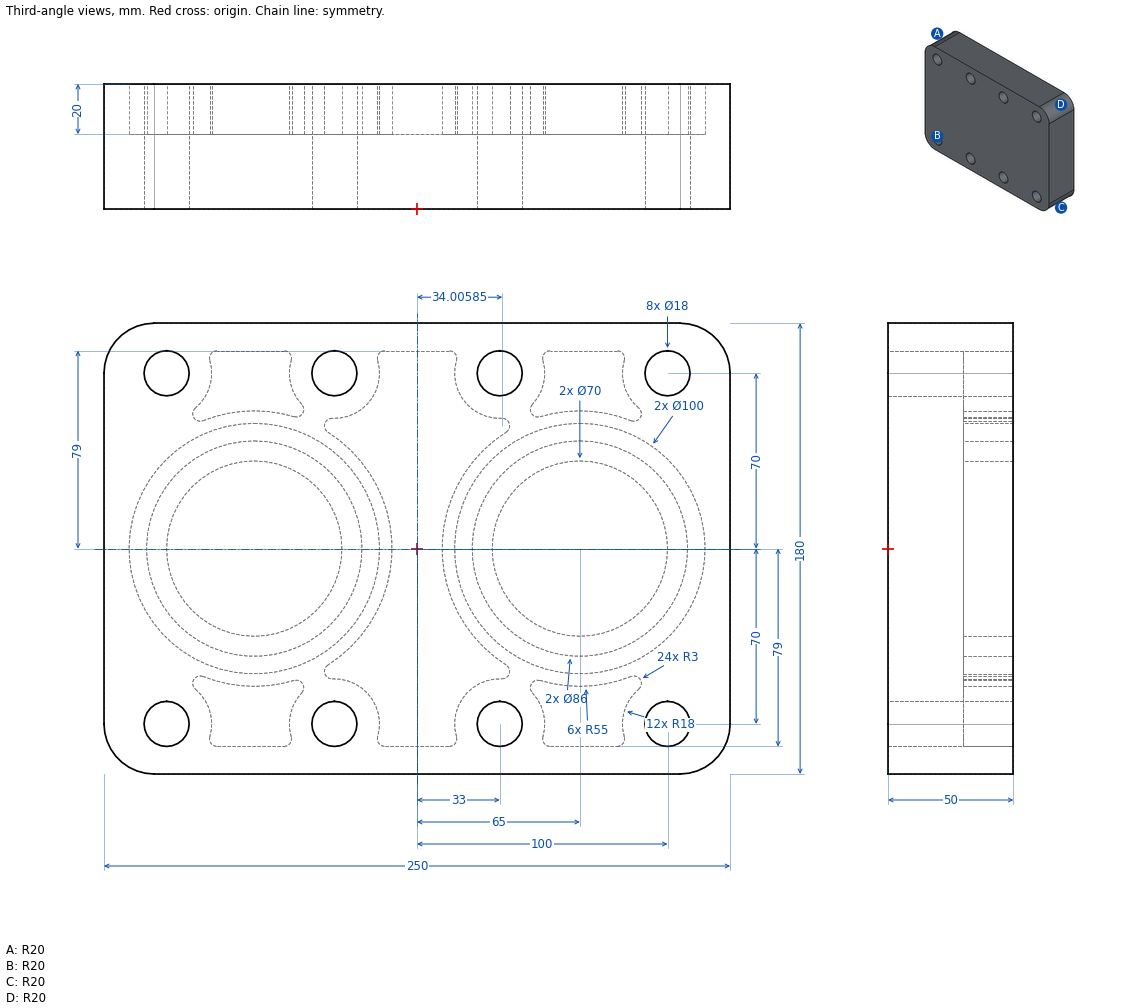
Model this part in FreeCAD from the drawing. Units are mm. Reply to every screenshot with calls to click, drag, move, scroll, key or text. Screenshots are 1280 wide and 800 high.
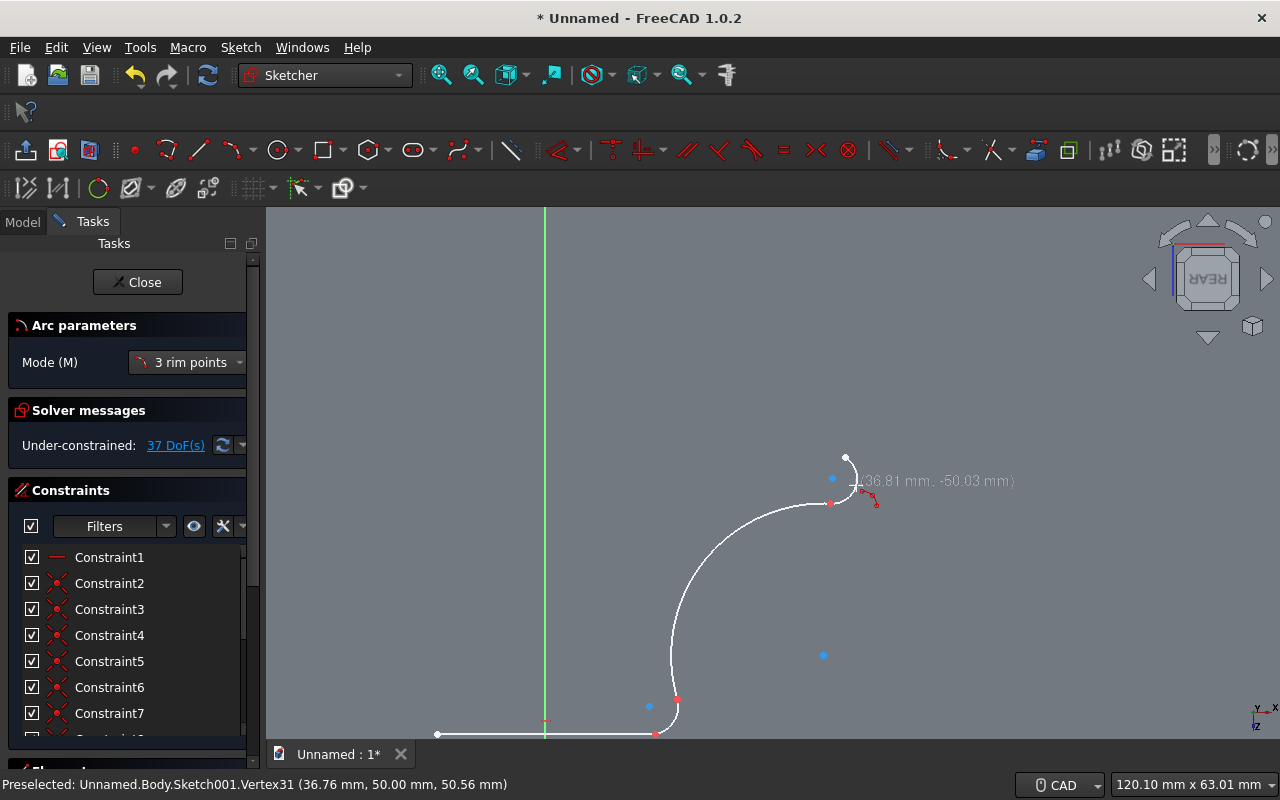
click(845, 457)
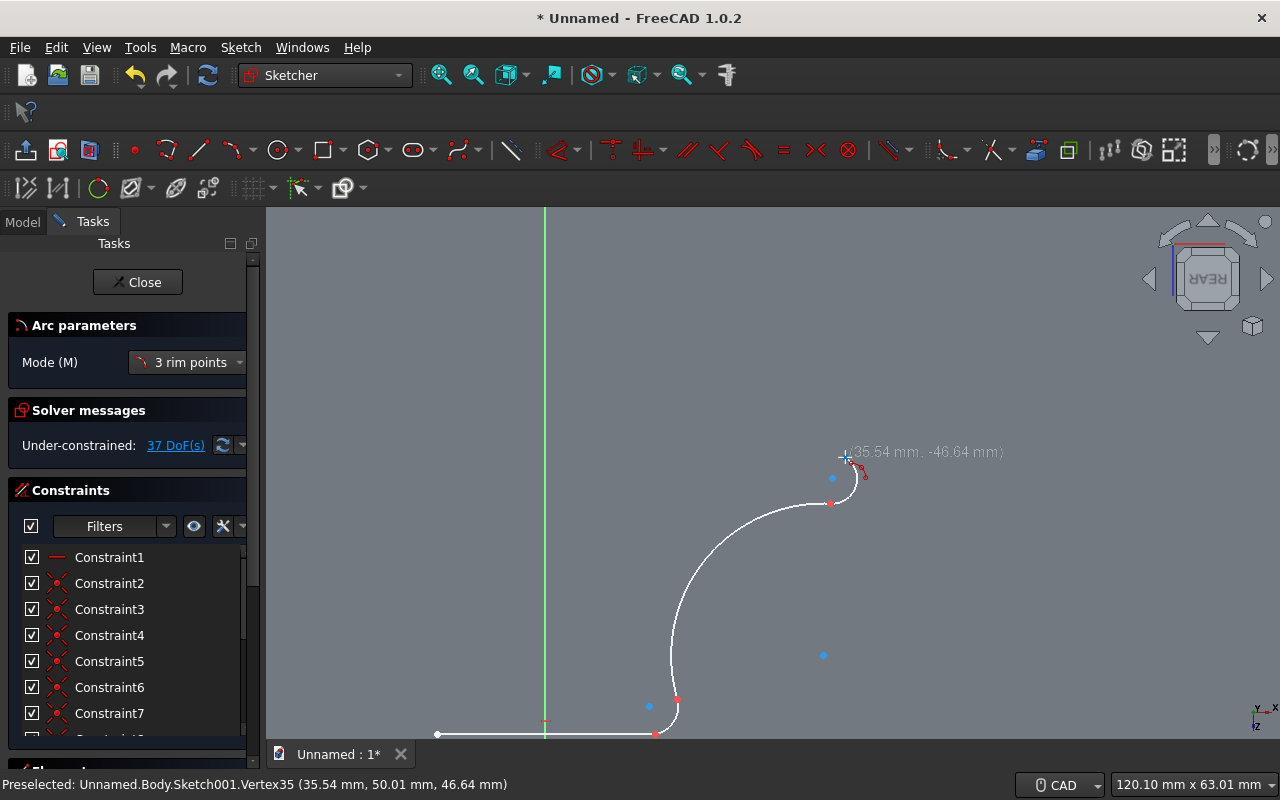
scroll(757, 607, down, 7)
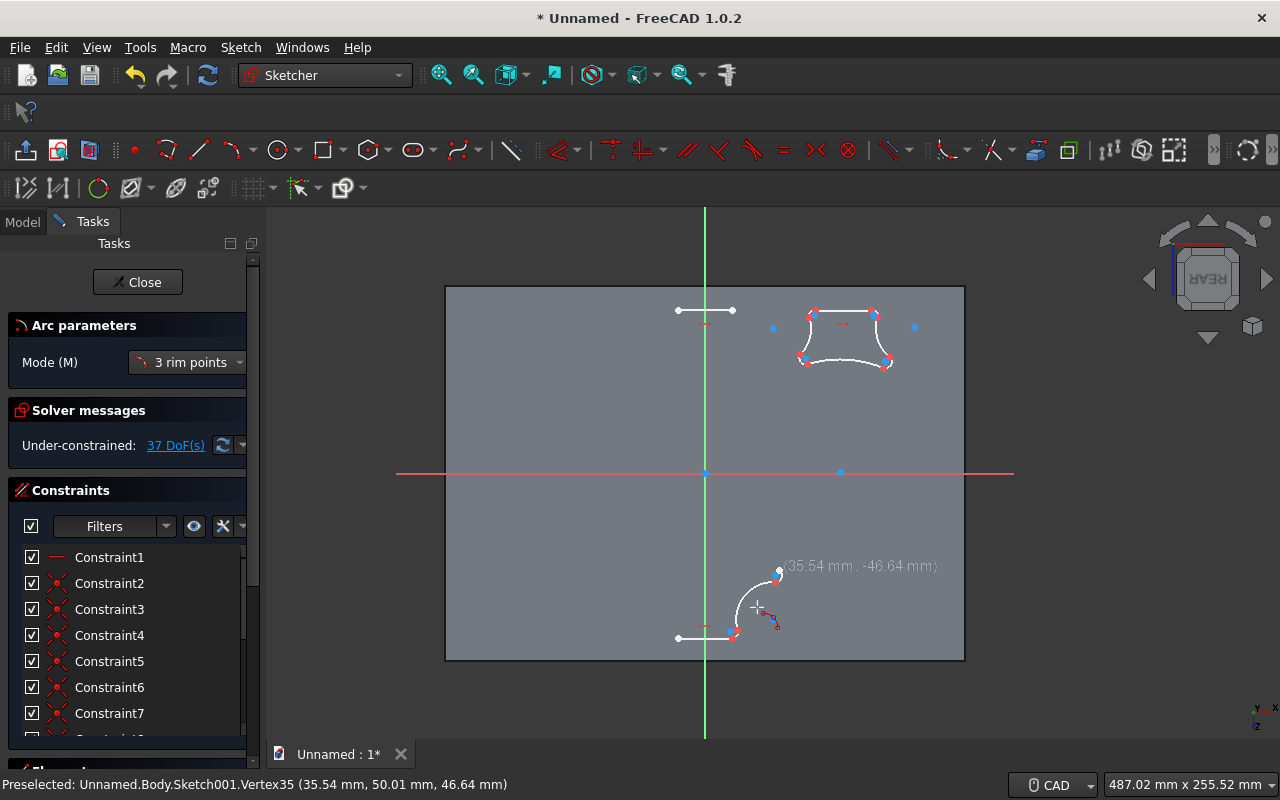
click(779, 377)
click(728, 451)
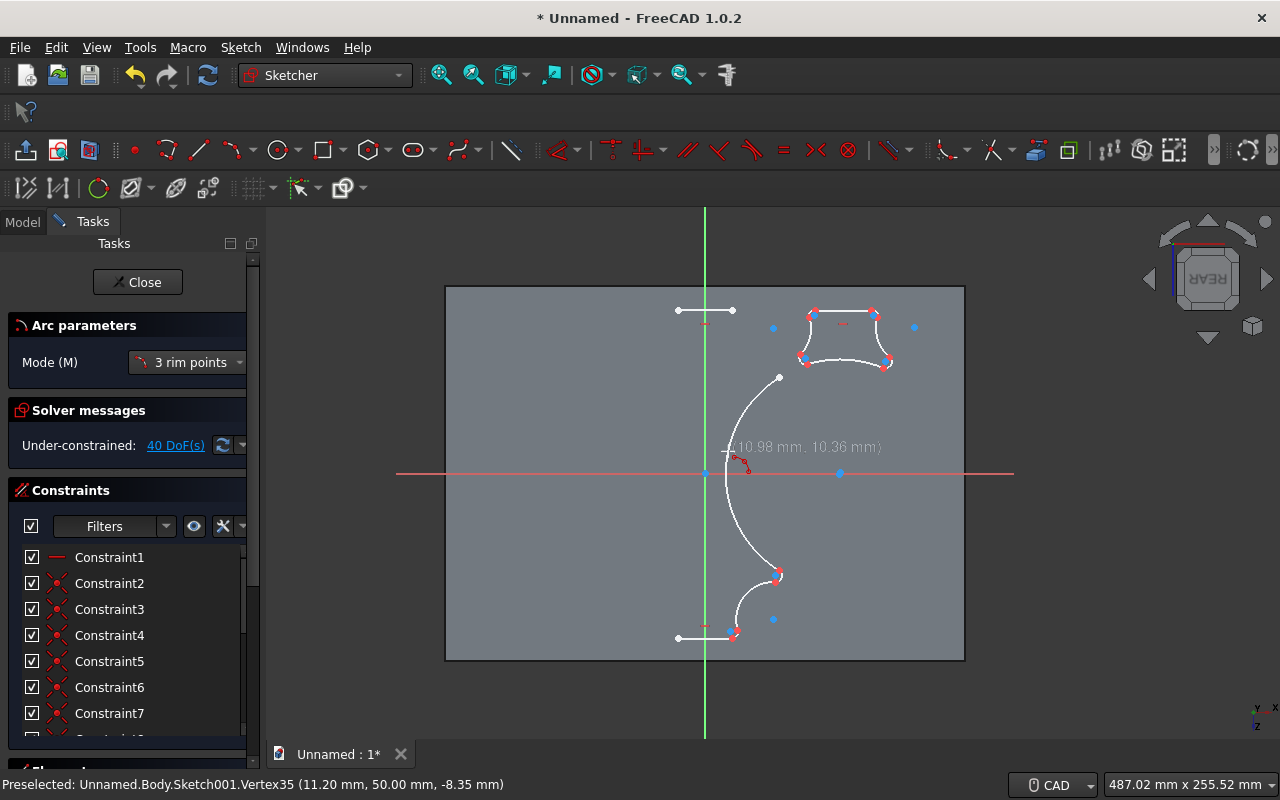
click(779, 378)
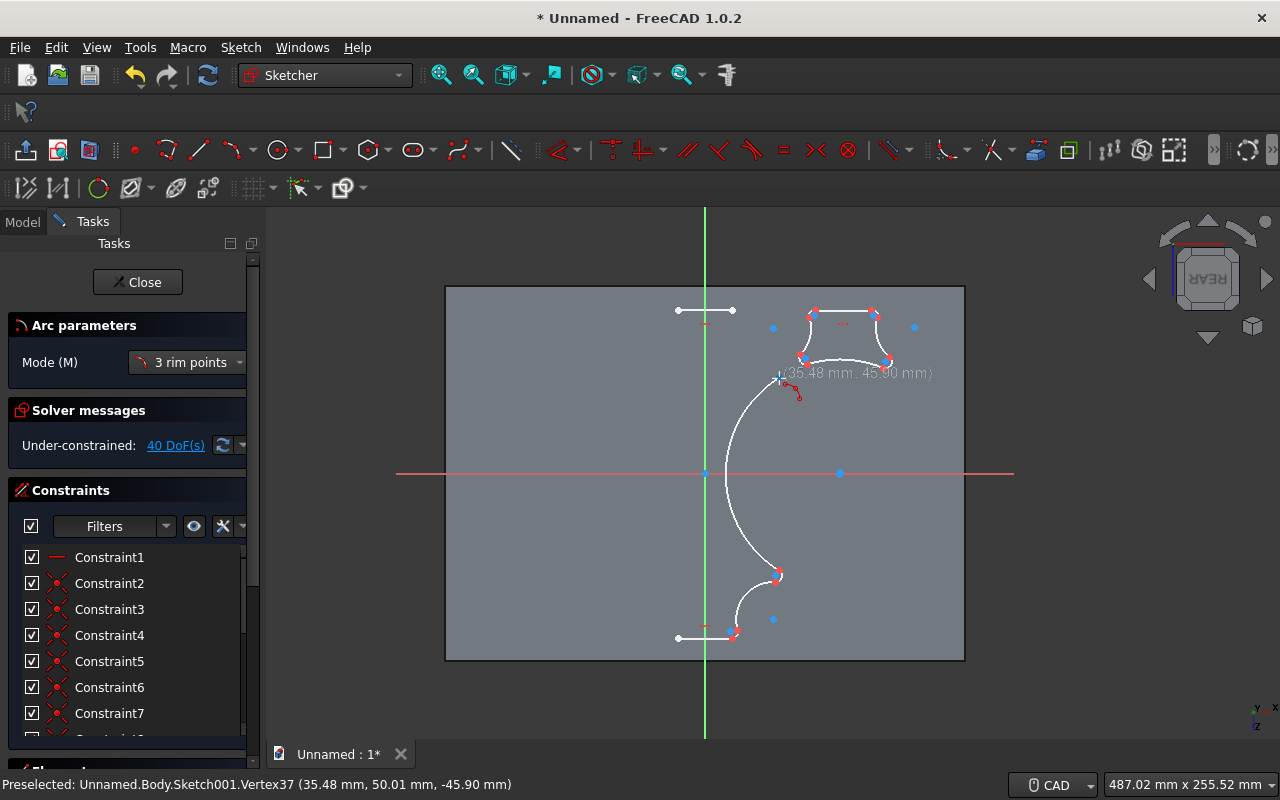
scroll(776, 365, up, 2)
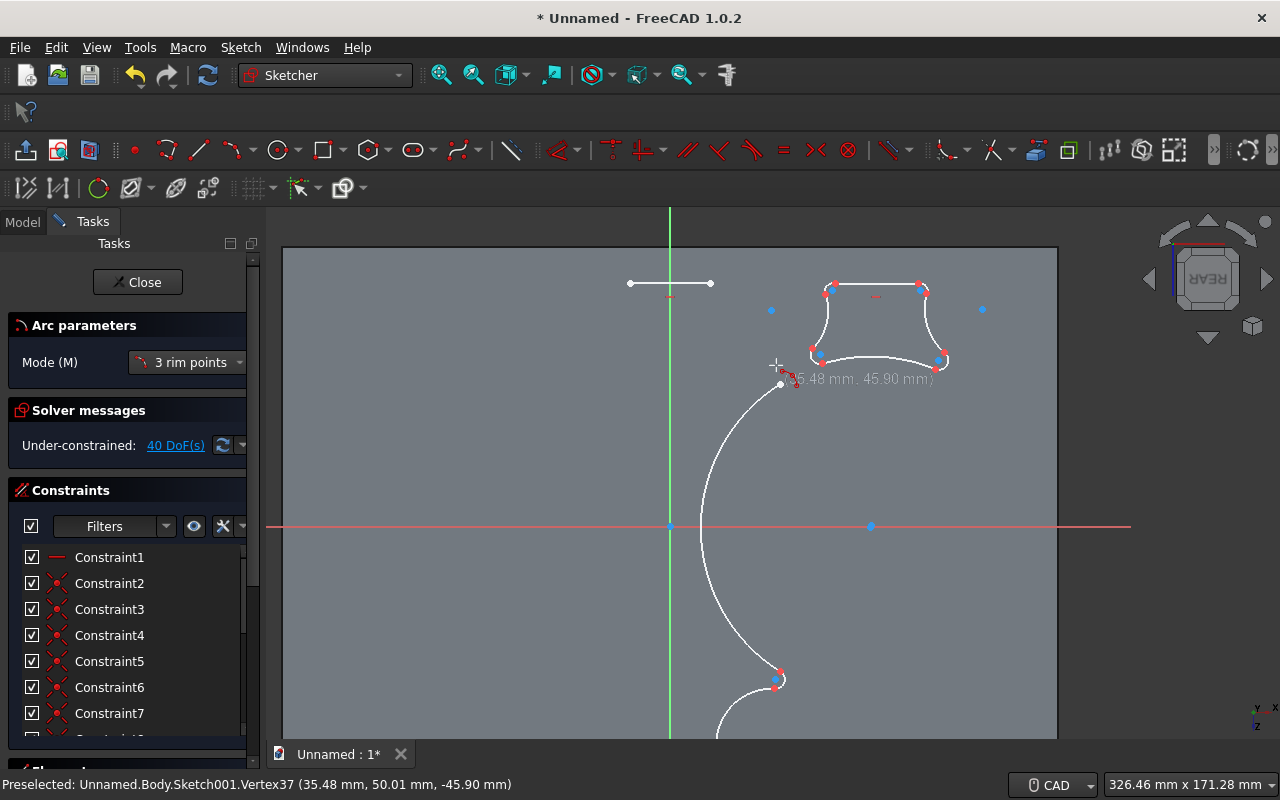
click(775, 365)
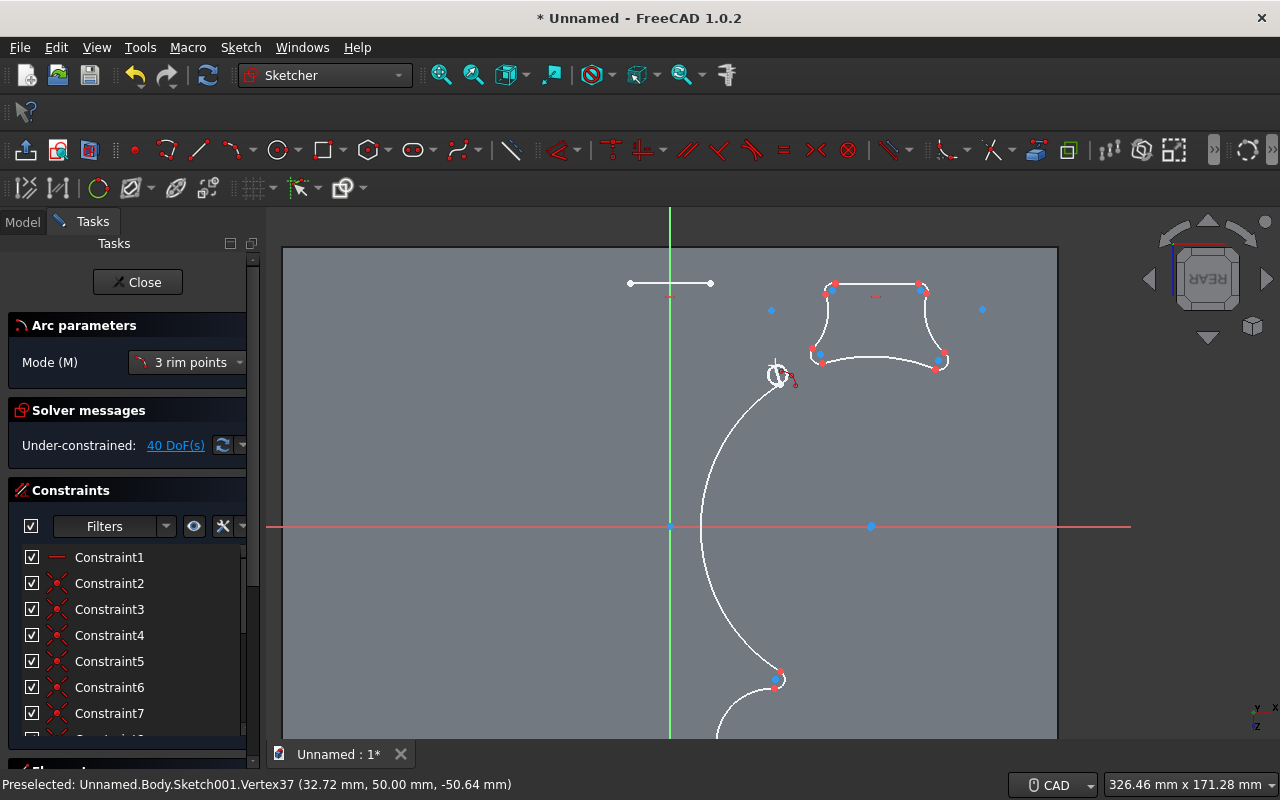
scroll(785, 372, up, 5)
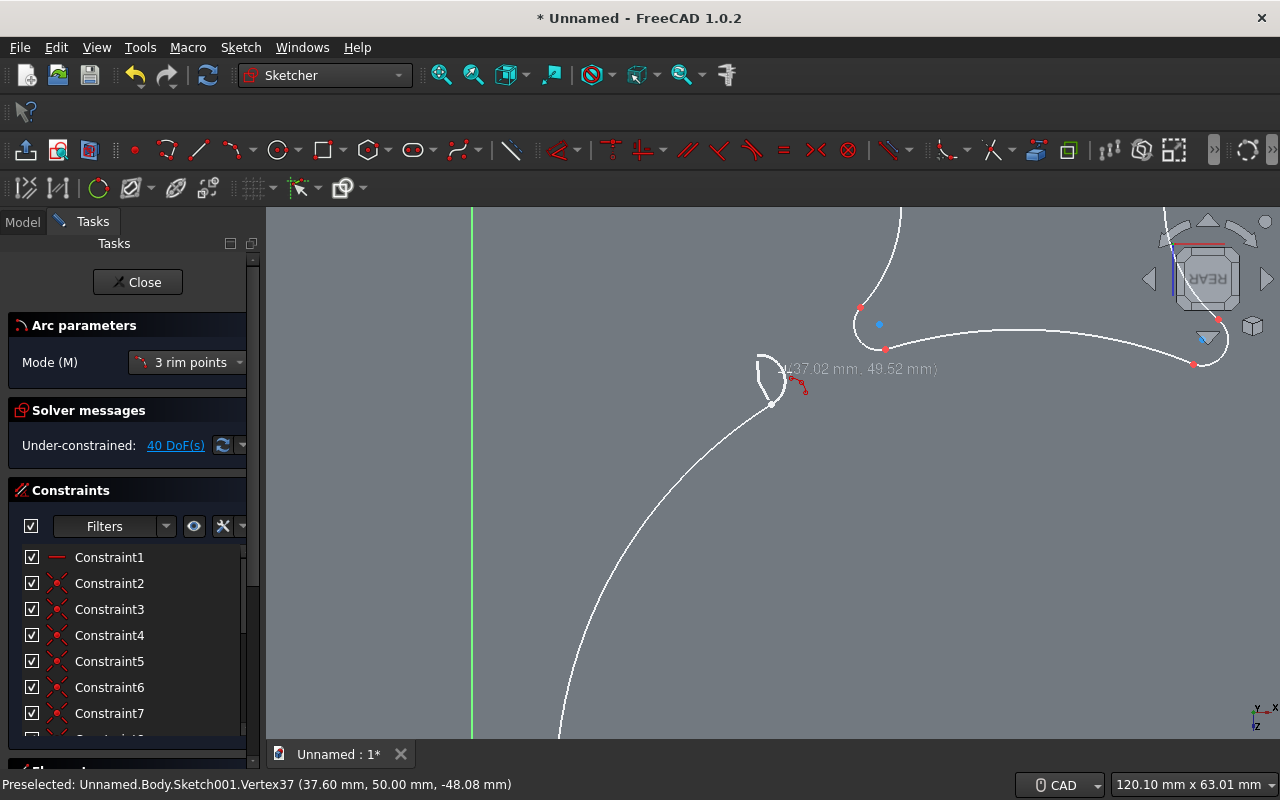
click(783, 371)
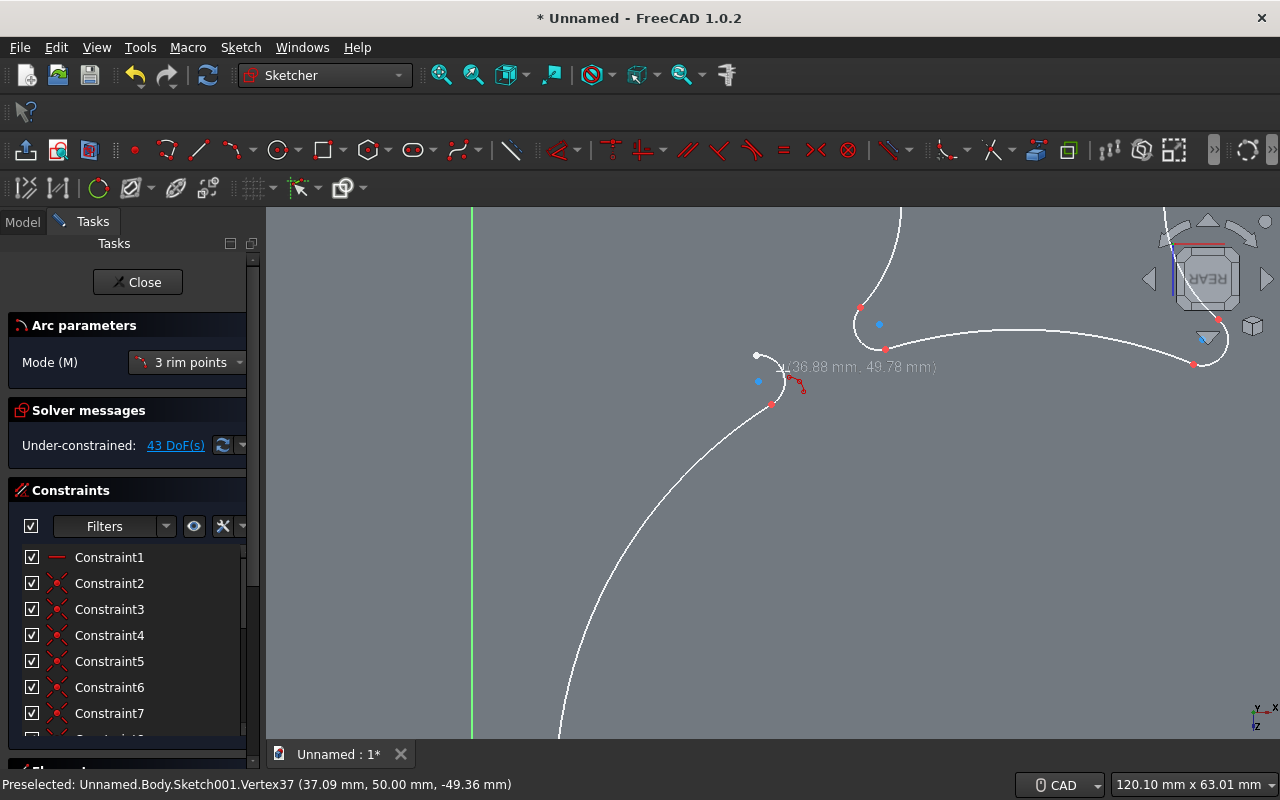
click(757, 355)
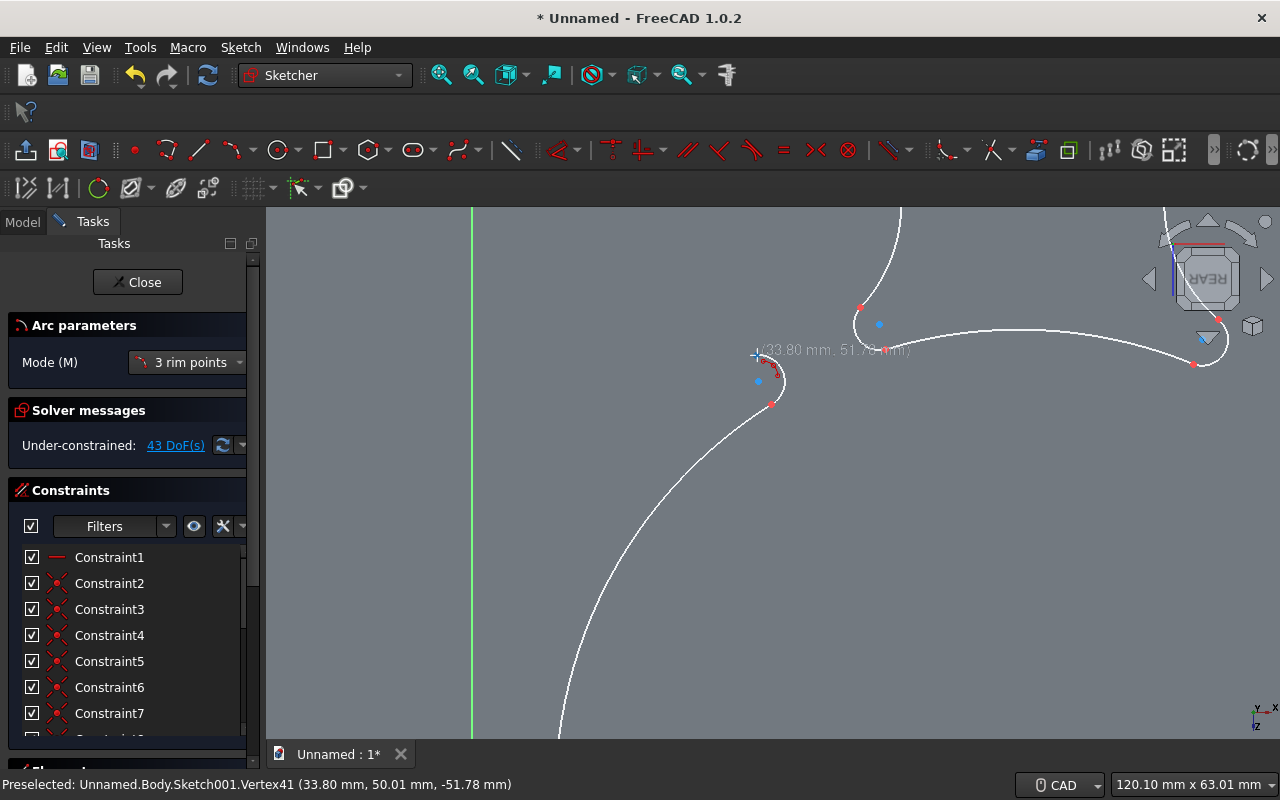
scroll(781, 368, down, 7)